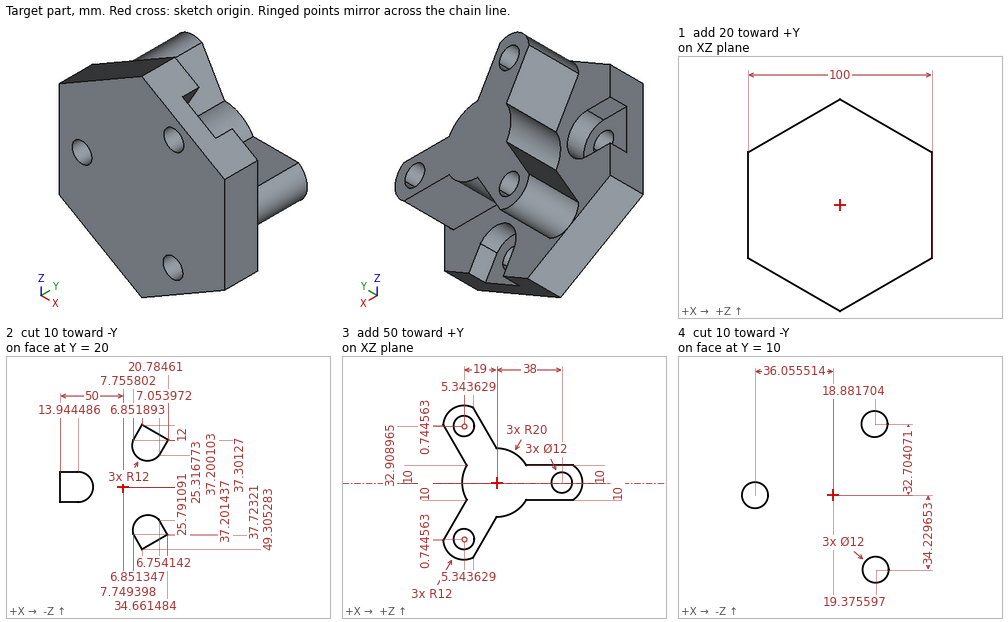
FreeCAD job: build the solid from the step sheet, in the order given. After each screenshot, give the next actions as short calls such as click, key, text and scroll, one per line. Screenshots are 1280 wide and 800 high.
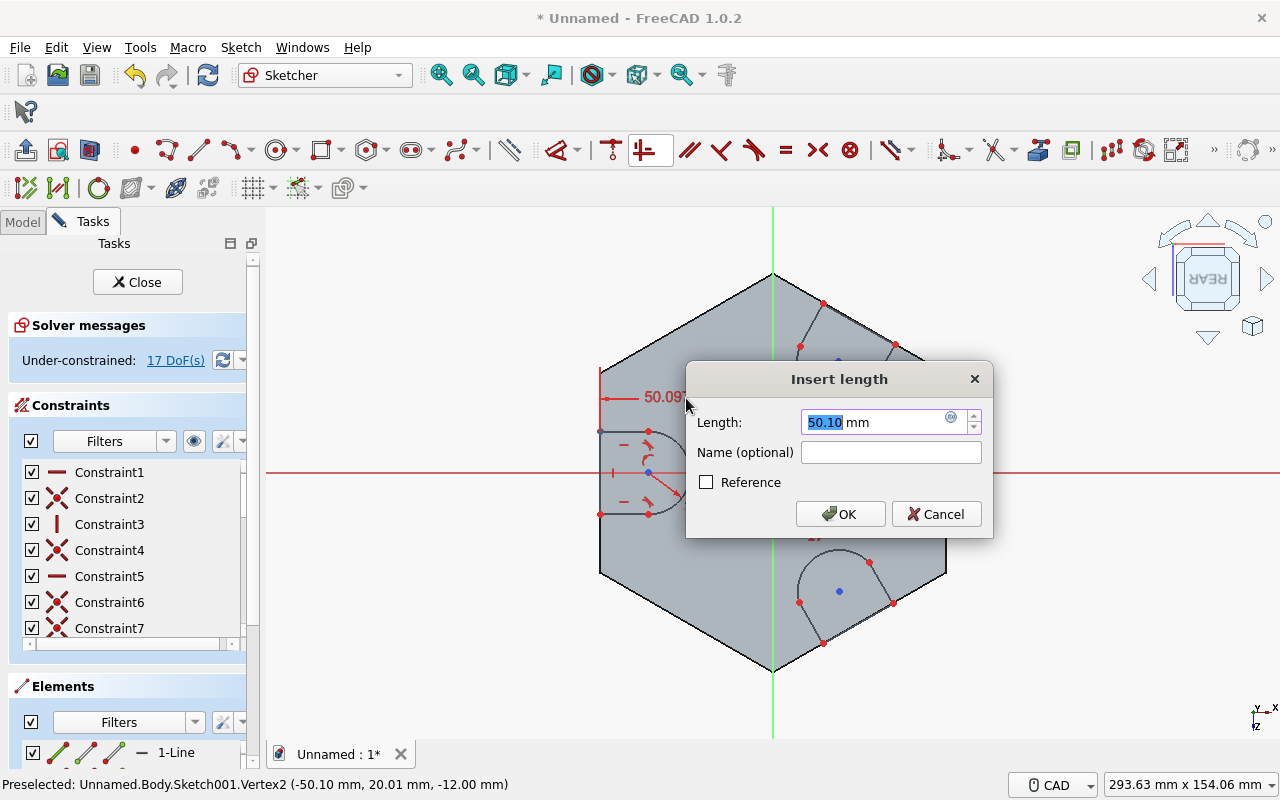
text(50)
key(Return)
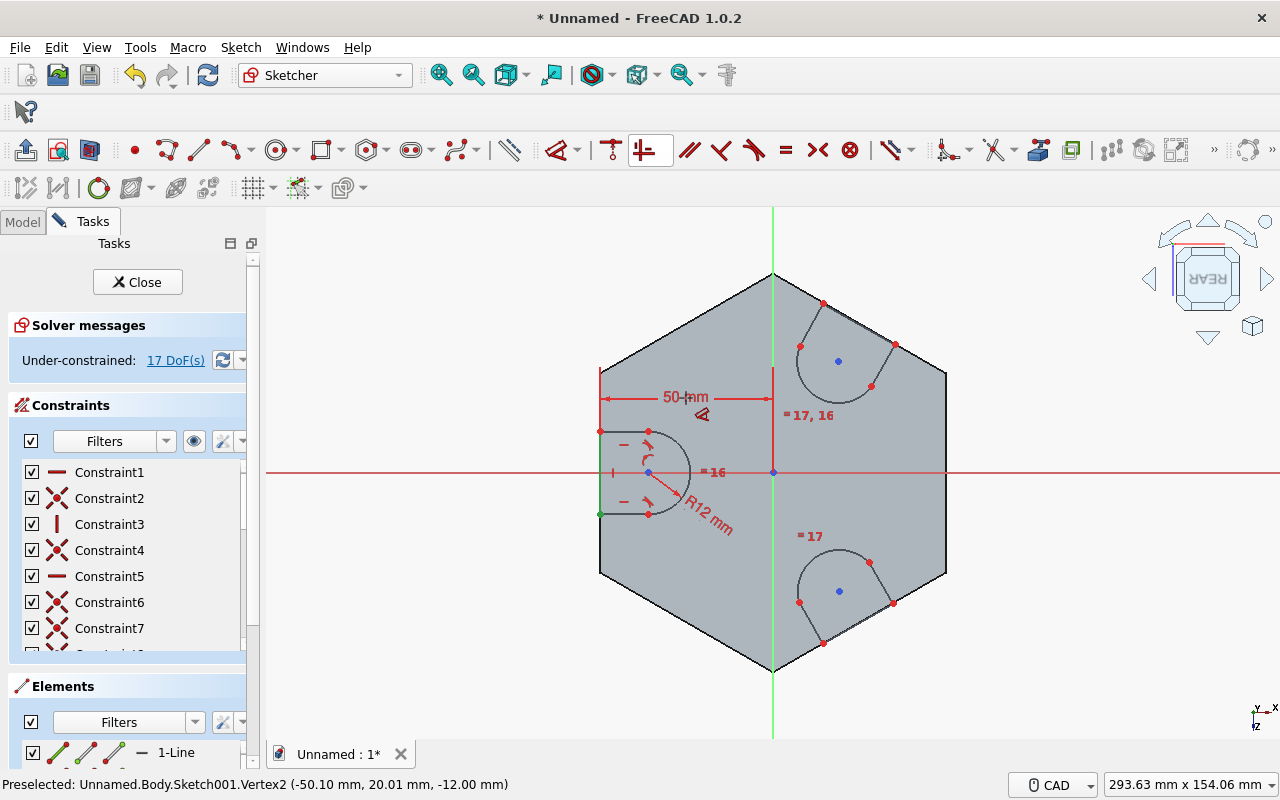
click(873, 333)
click(929, 325)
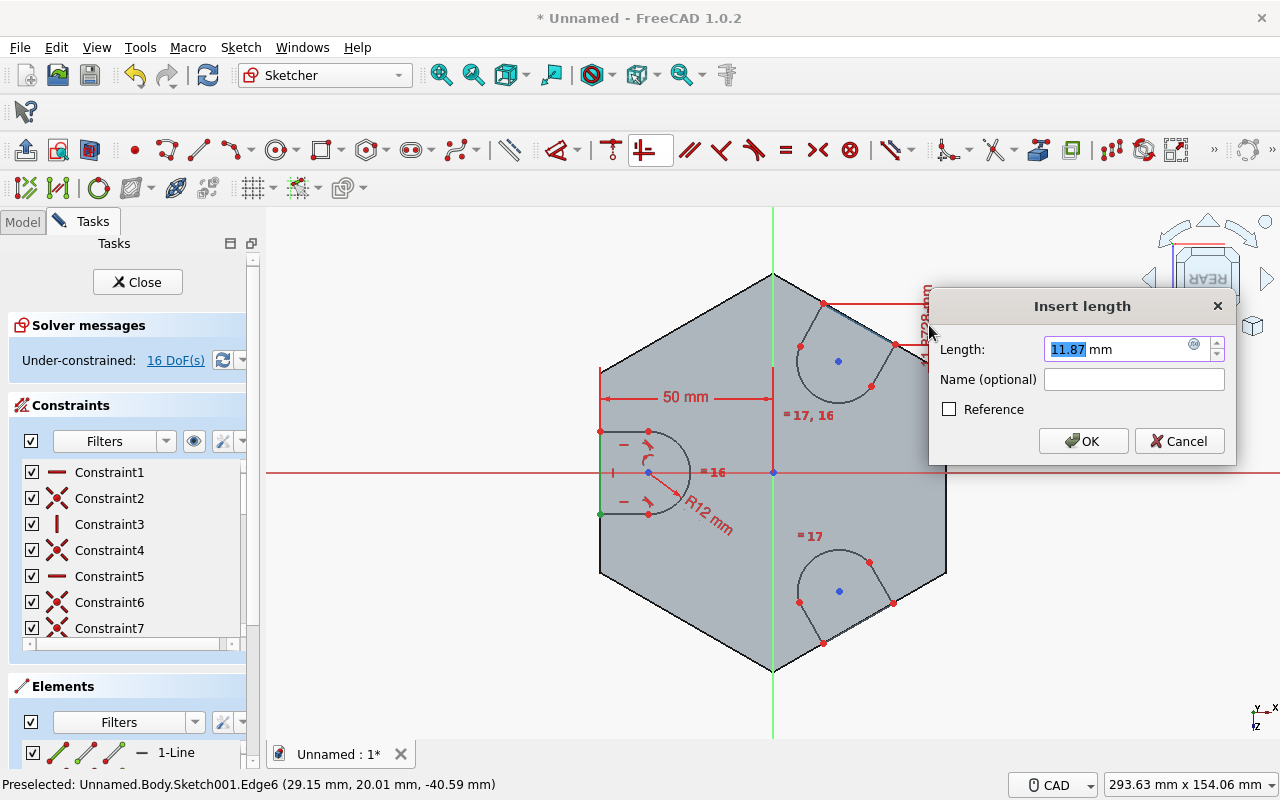
text(12)
key(Return)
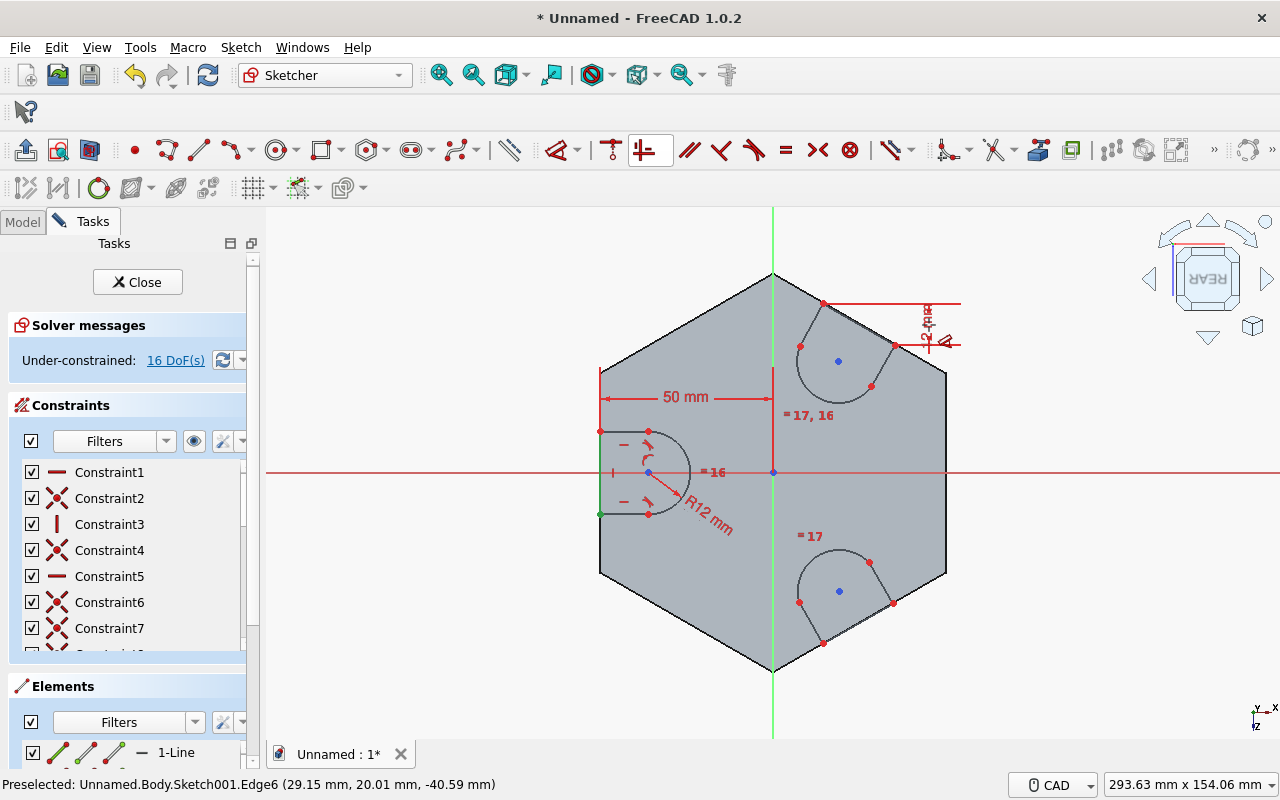
click(634, 432)
click(613, 398)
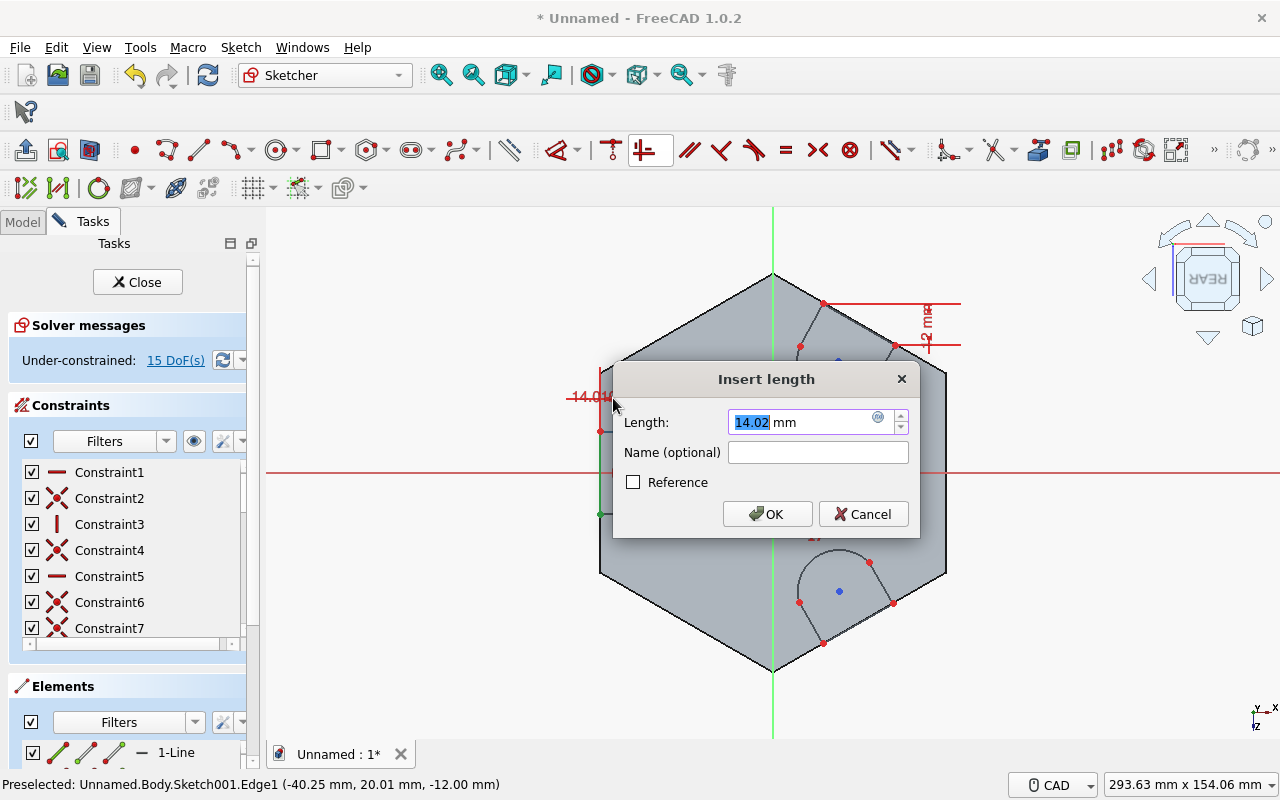
text(13.944486)
key(Return)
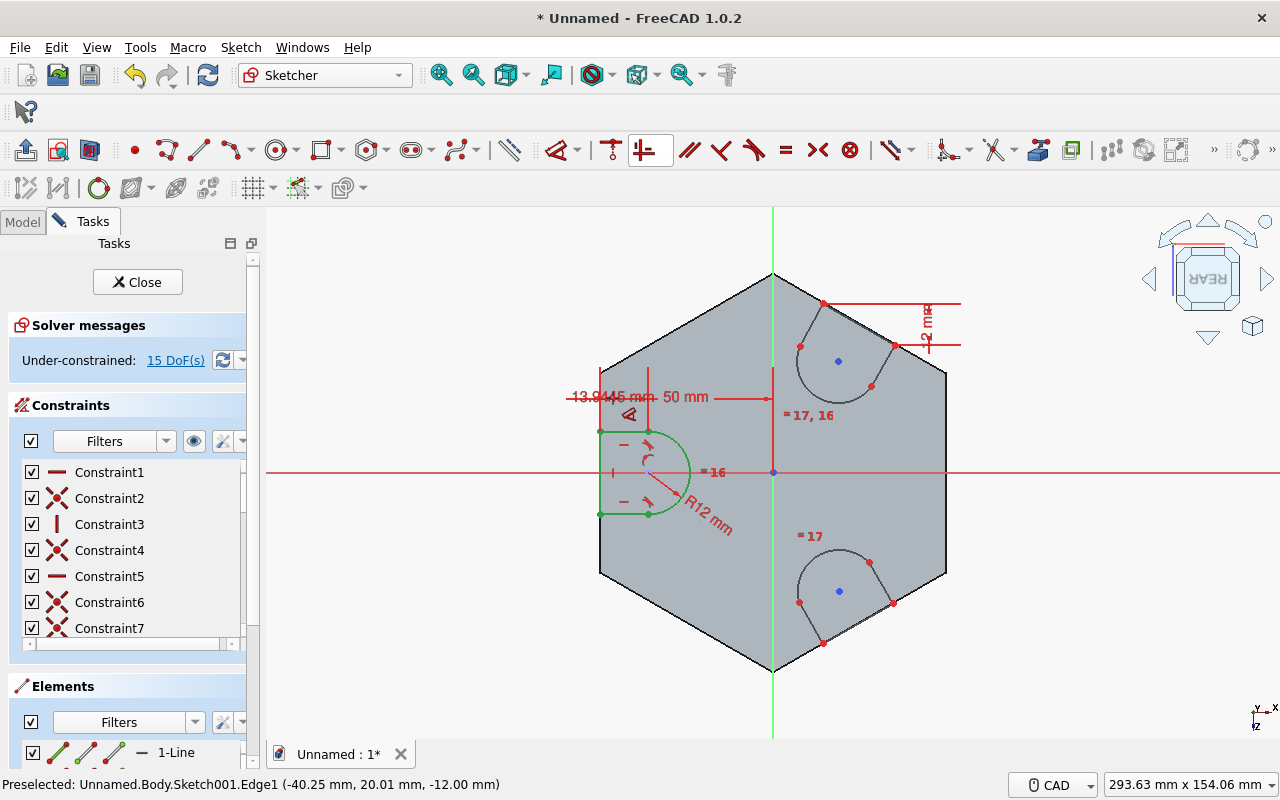
click(895, 345)
click(929, 409)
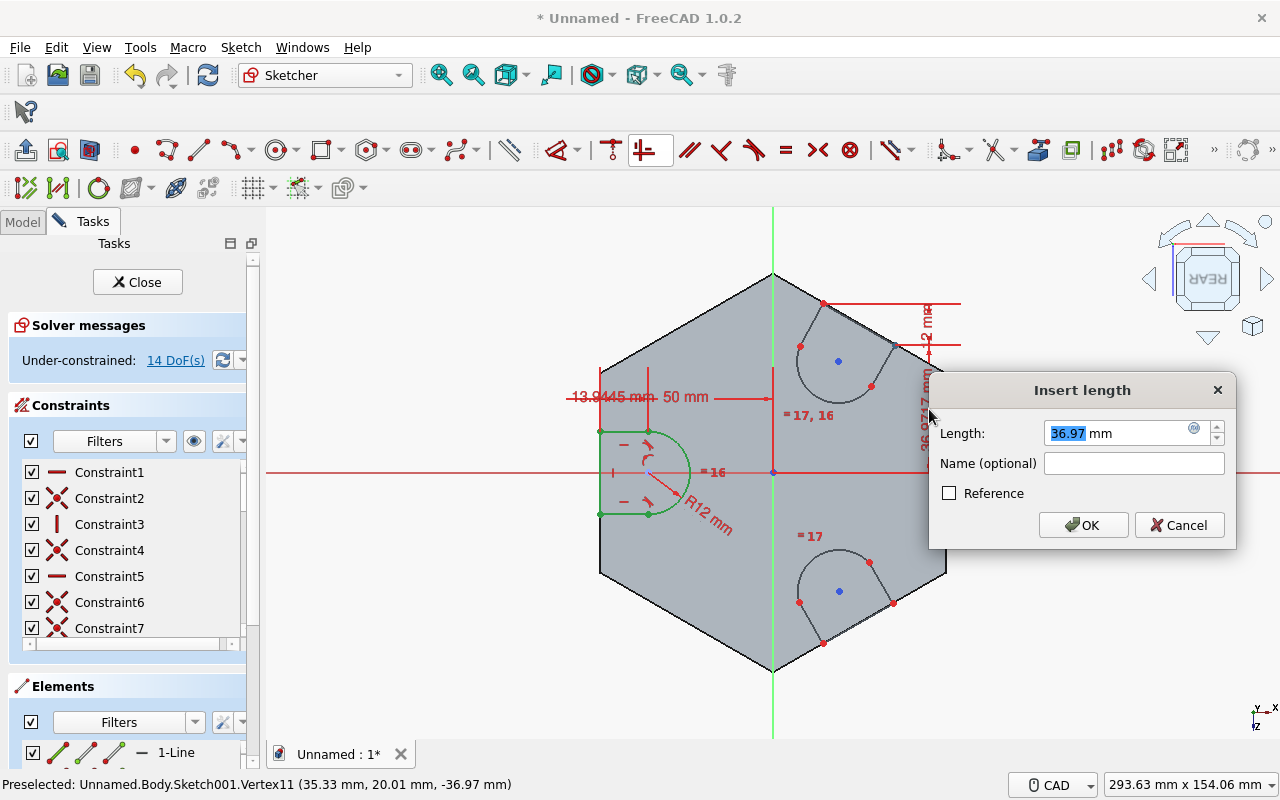
text(37.30127)
key(Return)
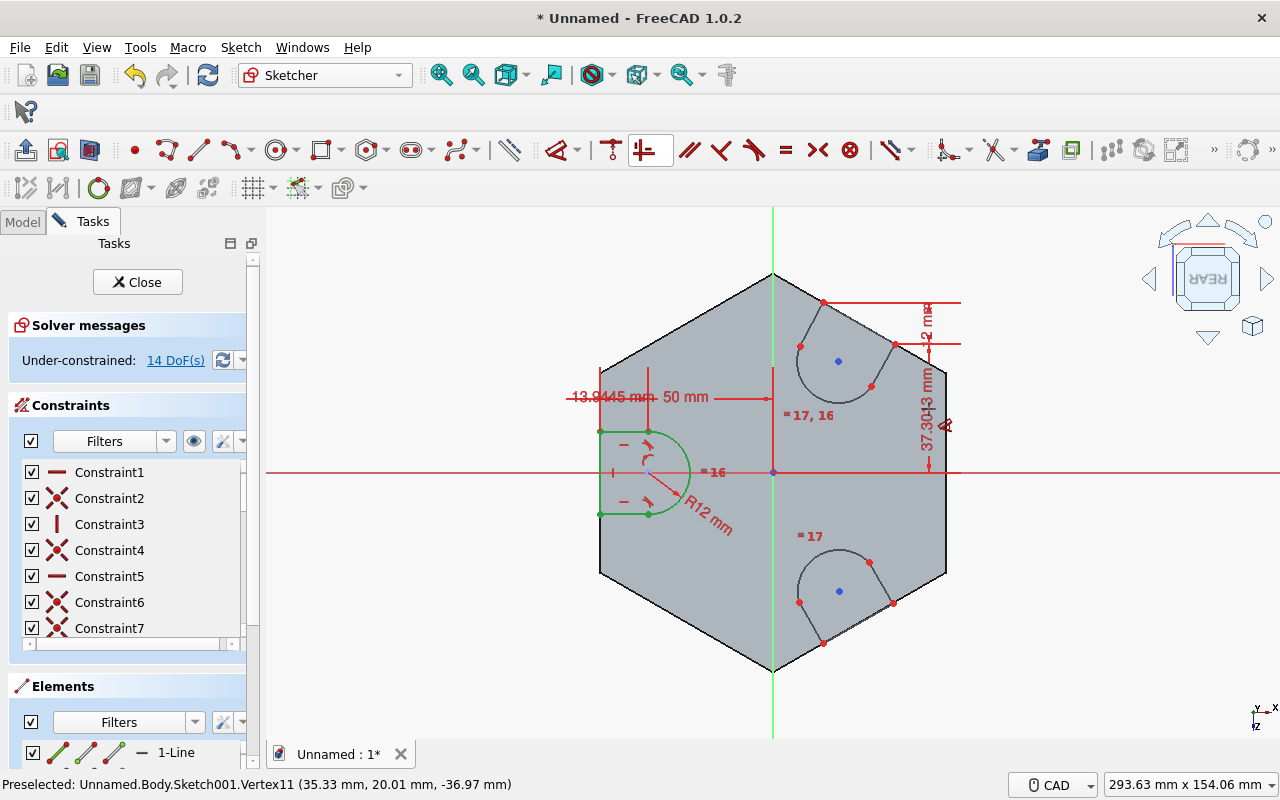
scroll(800, 346, up, 2)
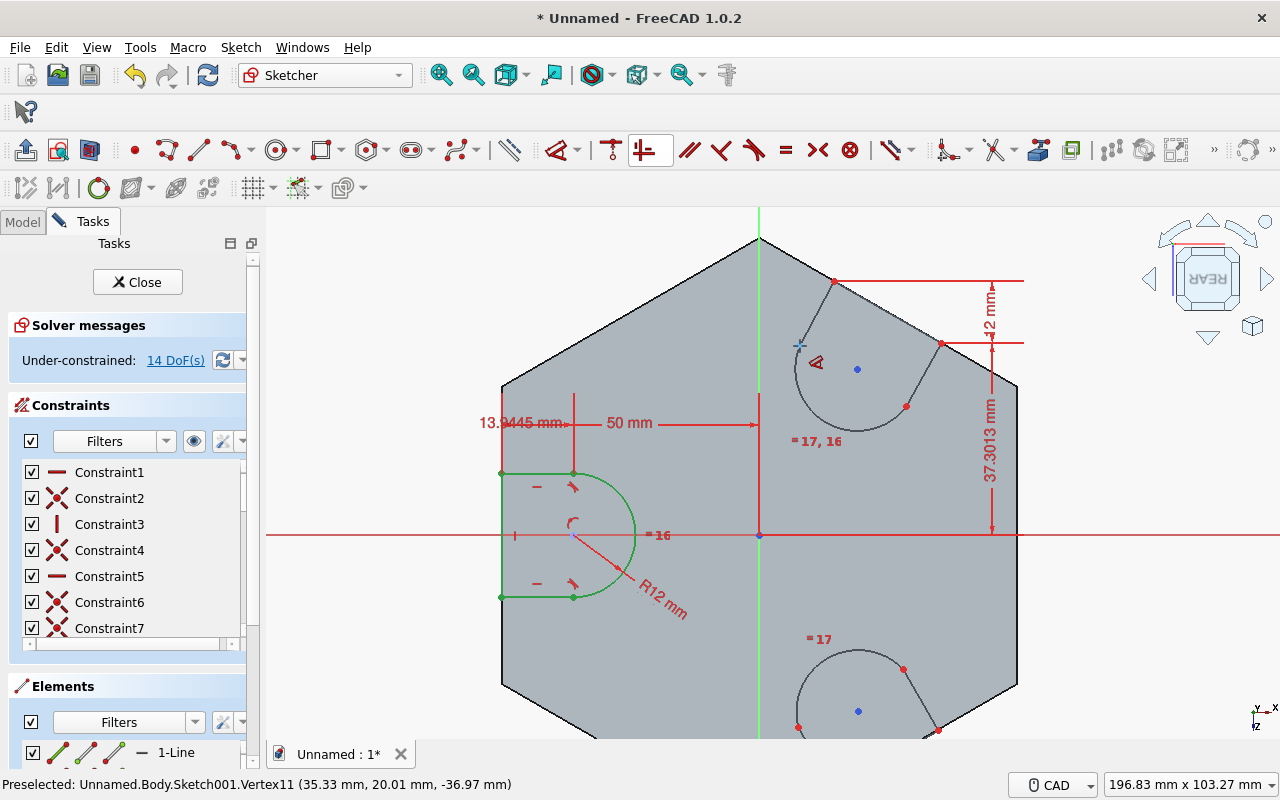
click(800, 346)
click(780, 312)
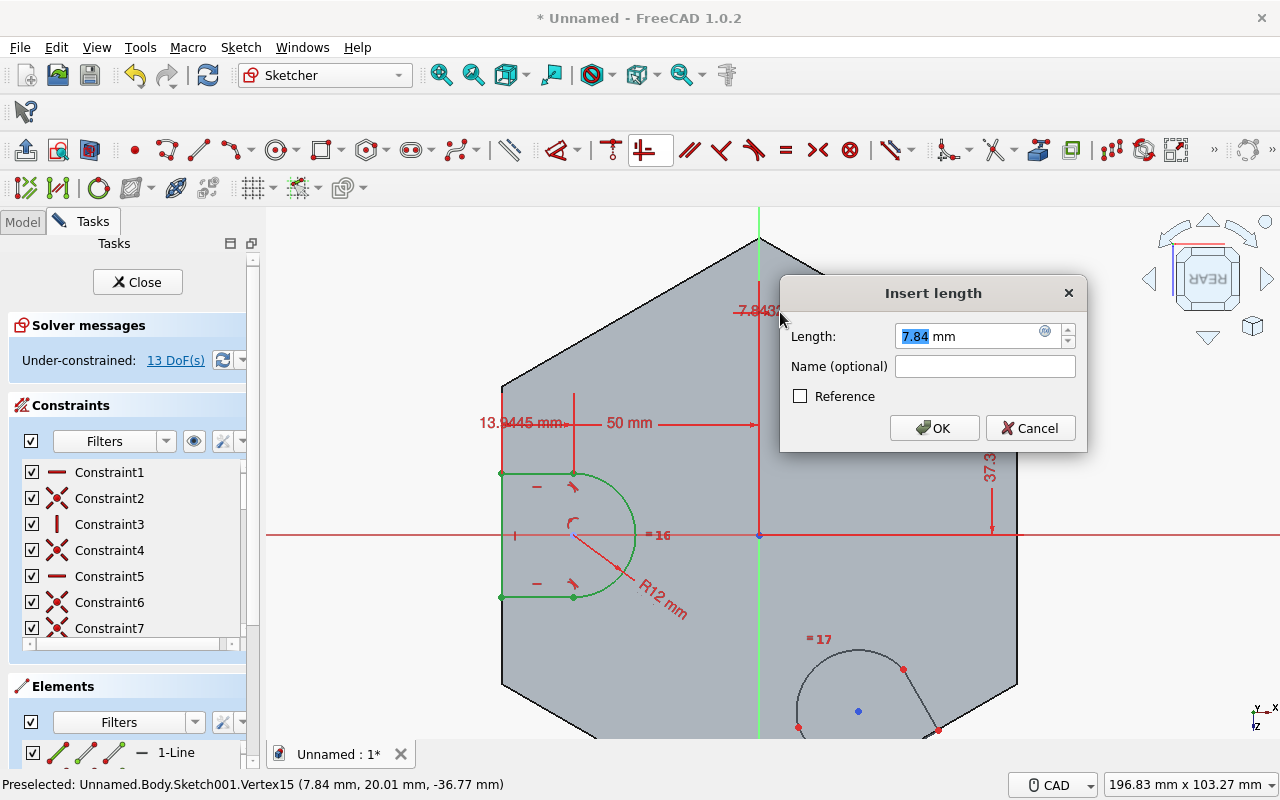
text(7.755802)
key(Return)